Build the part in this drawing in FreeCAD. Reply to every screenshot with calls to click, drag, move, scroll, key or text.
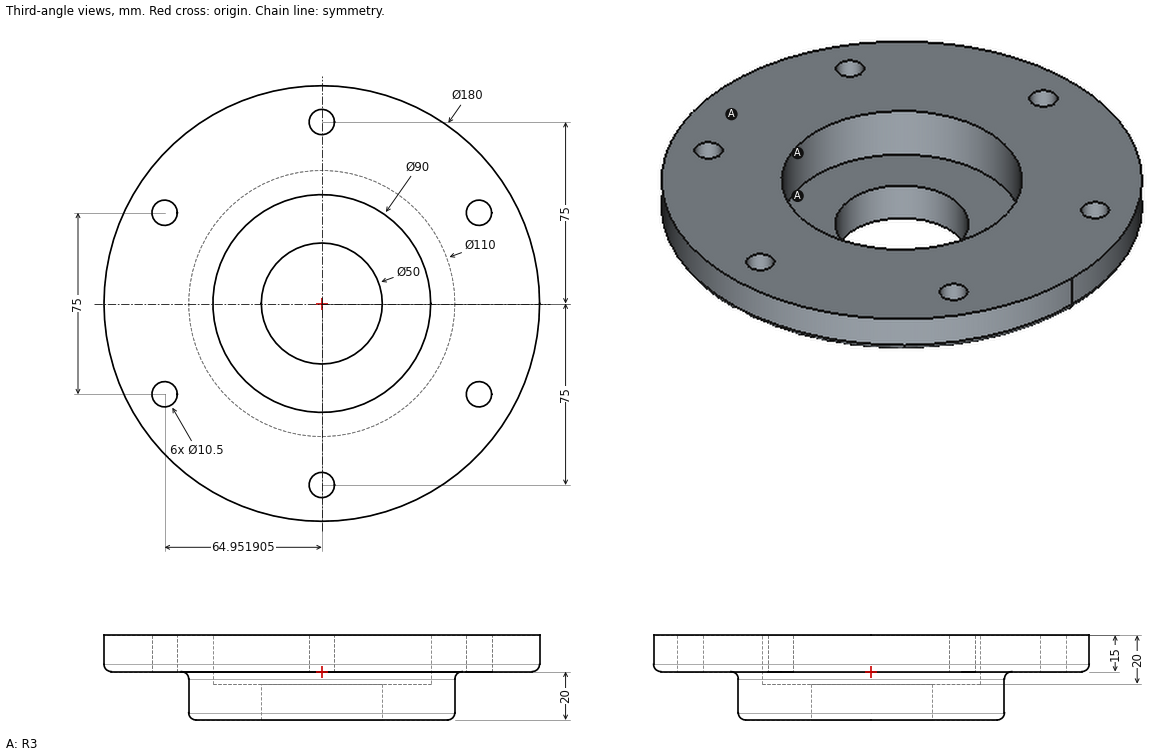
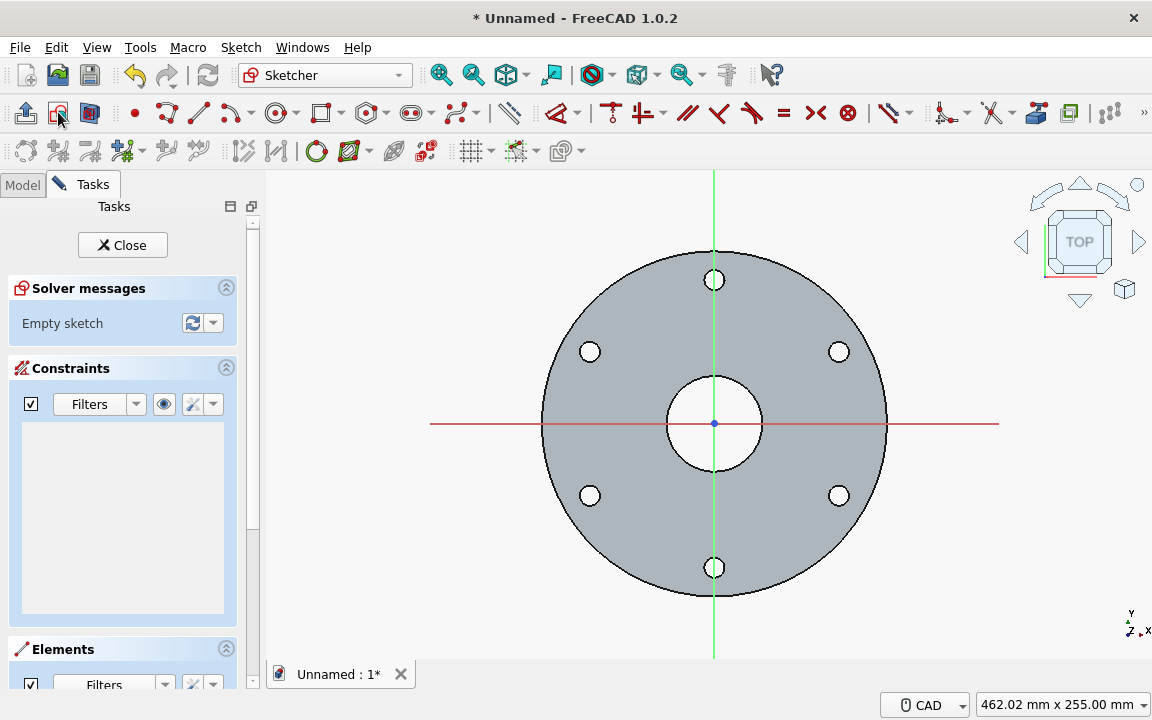
scroll(804, 435, up, 3)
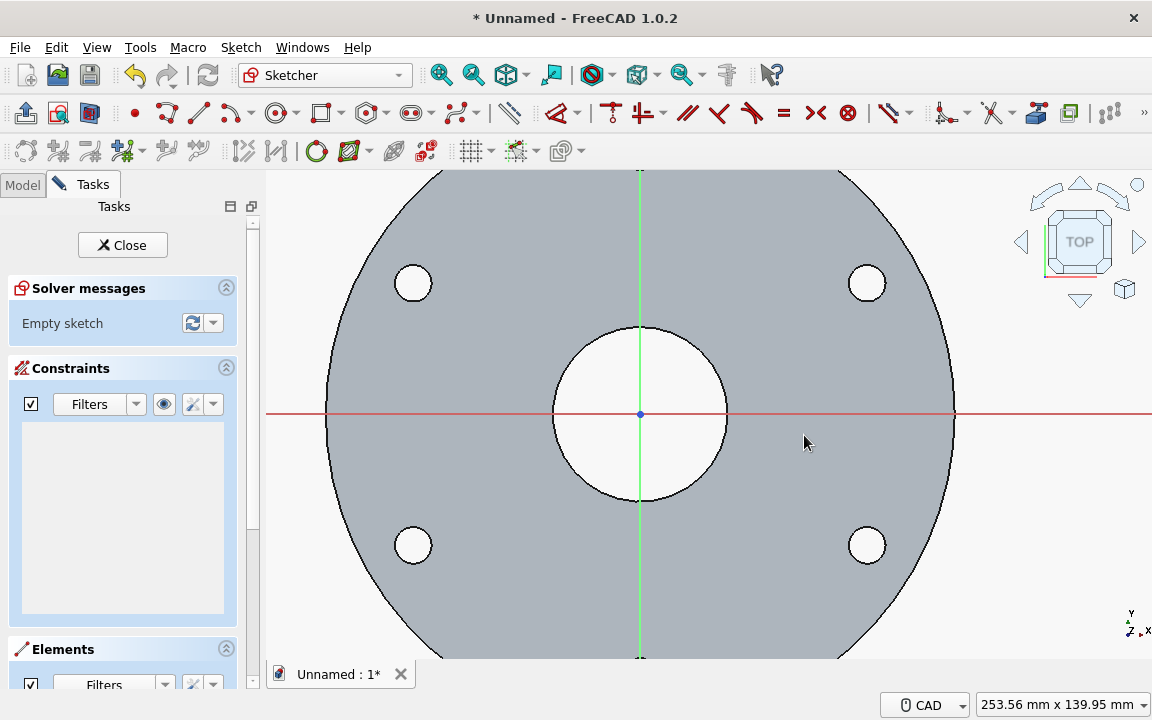
key(g)
key(c)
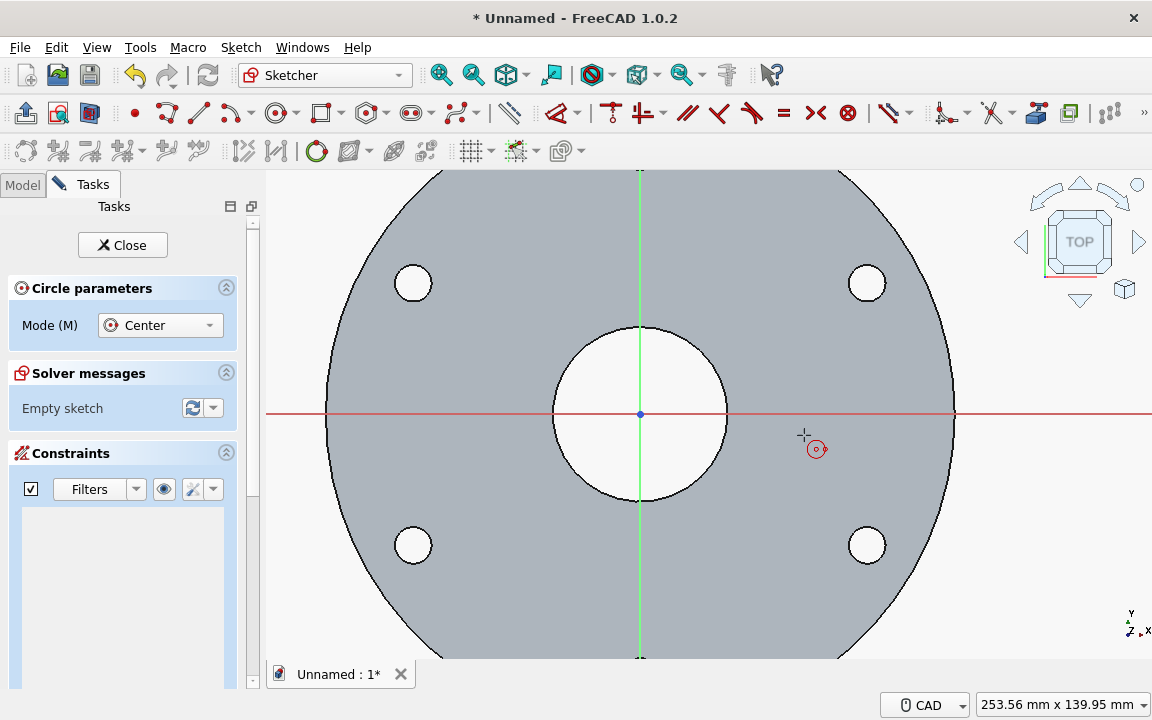
click(640, 414)
move(751, 303)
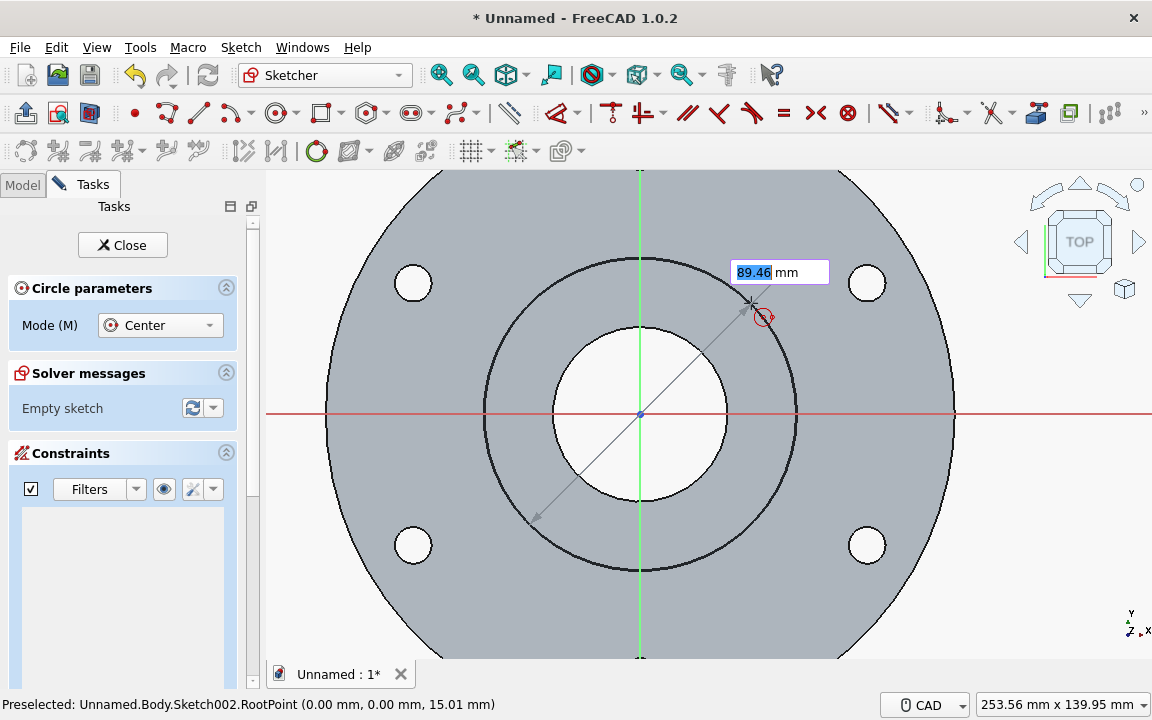
text(90)
key(Return)
key(Escape)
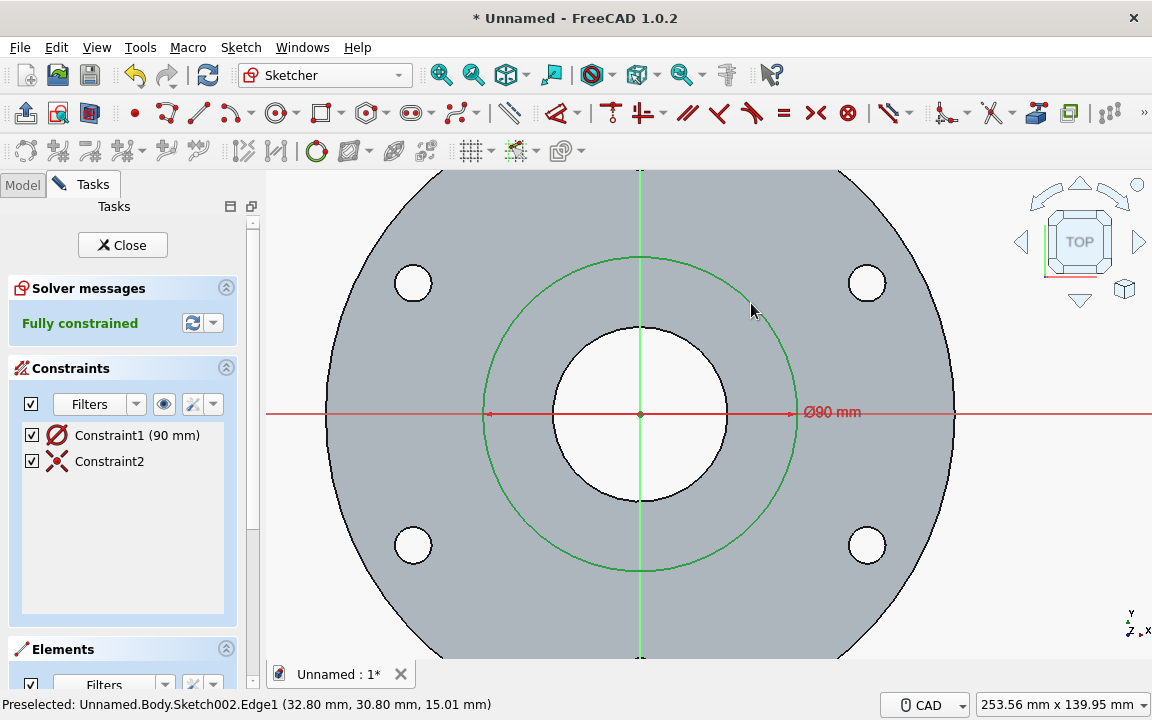
click(123, 245)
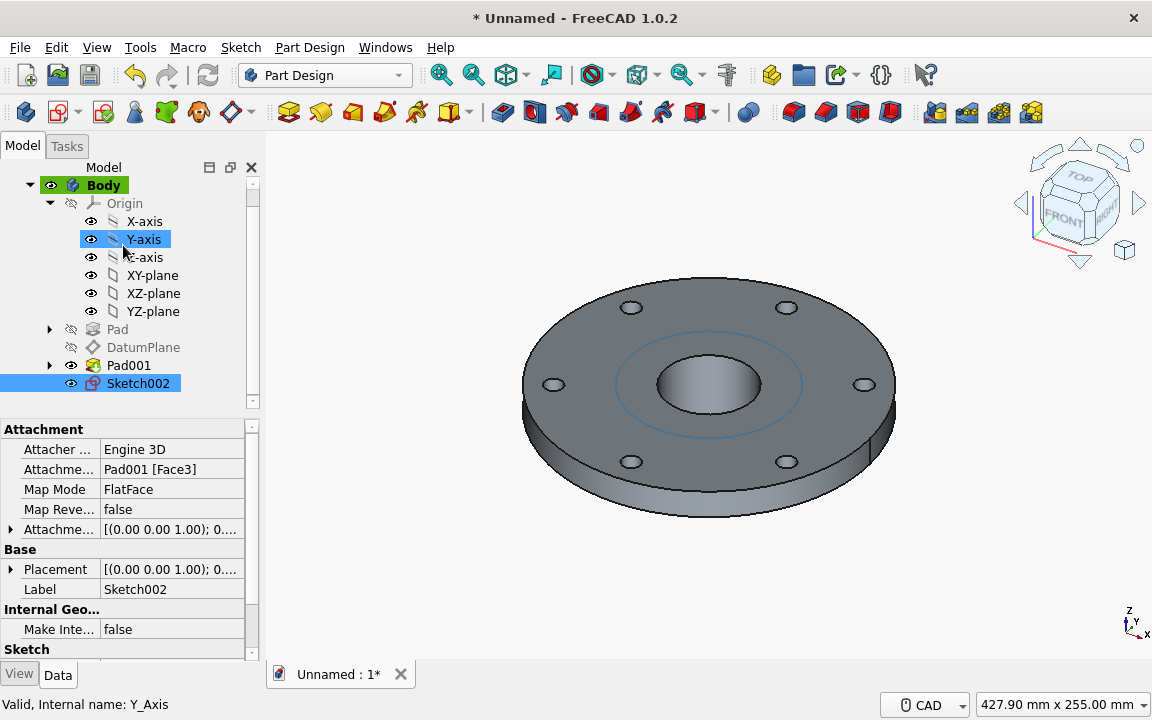
click(504, 112)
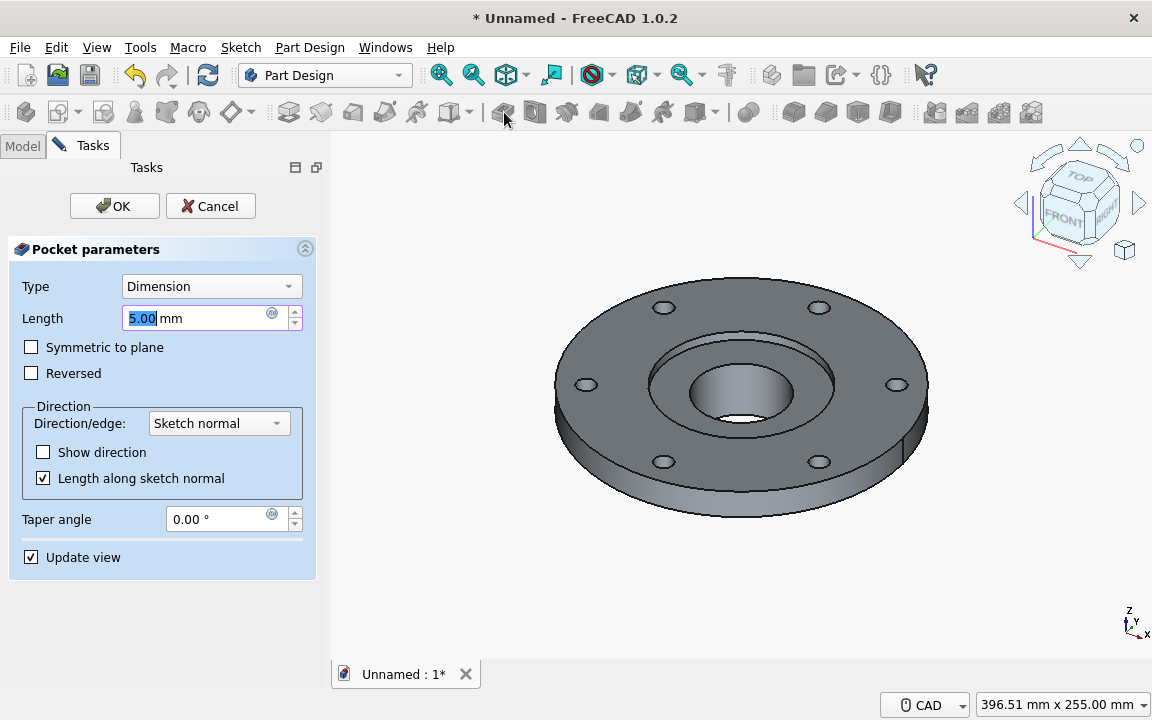
text(20)
key(Tab)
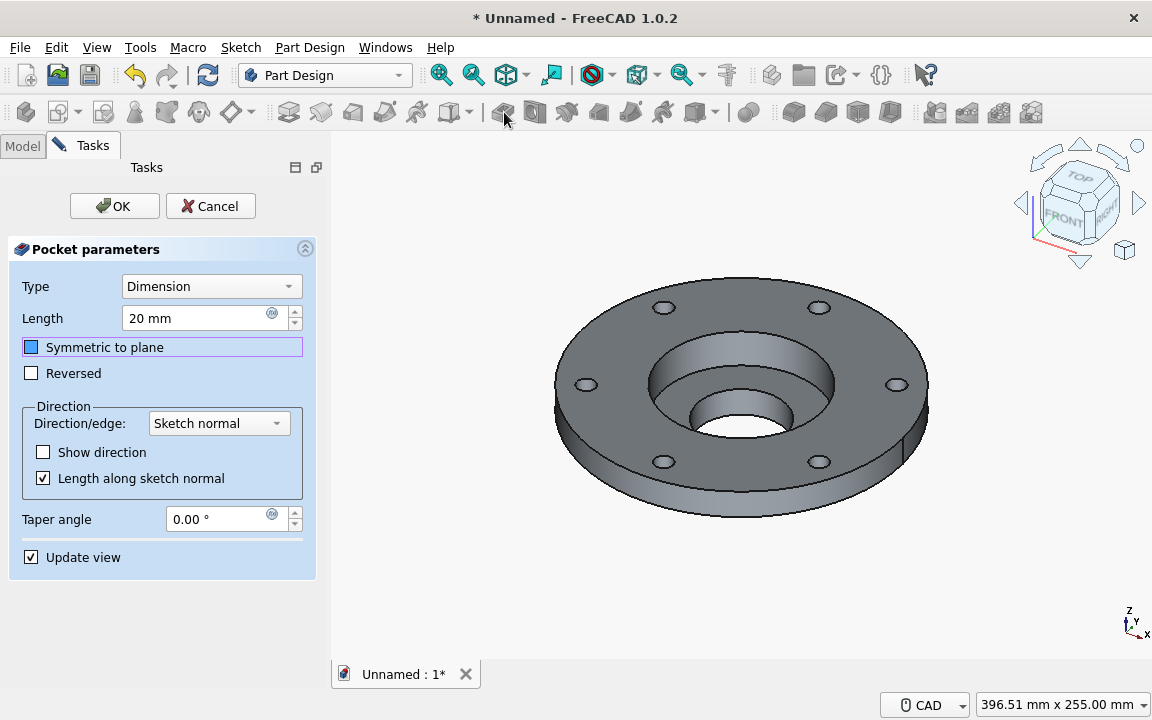
click(115, 206)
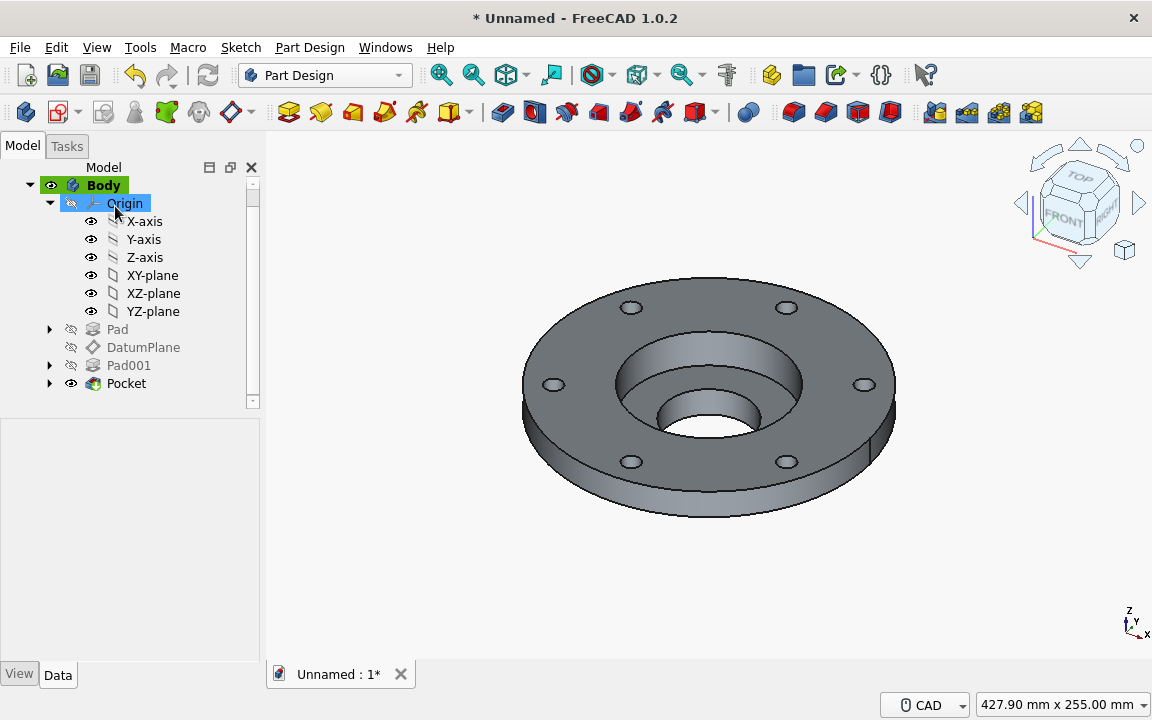
key(0)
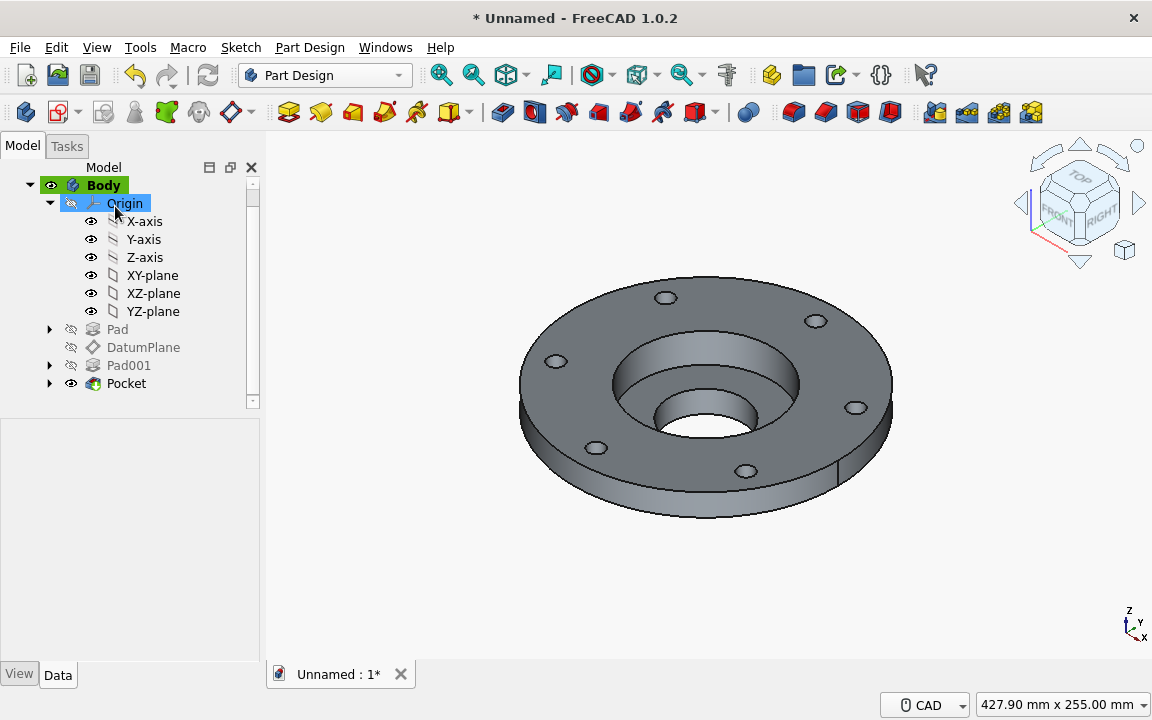
key(2)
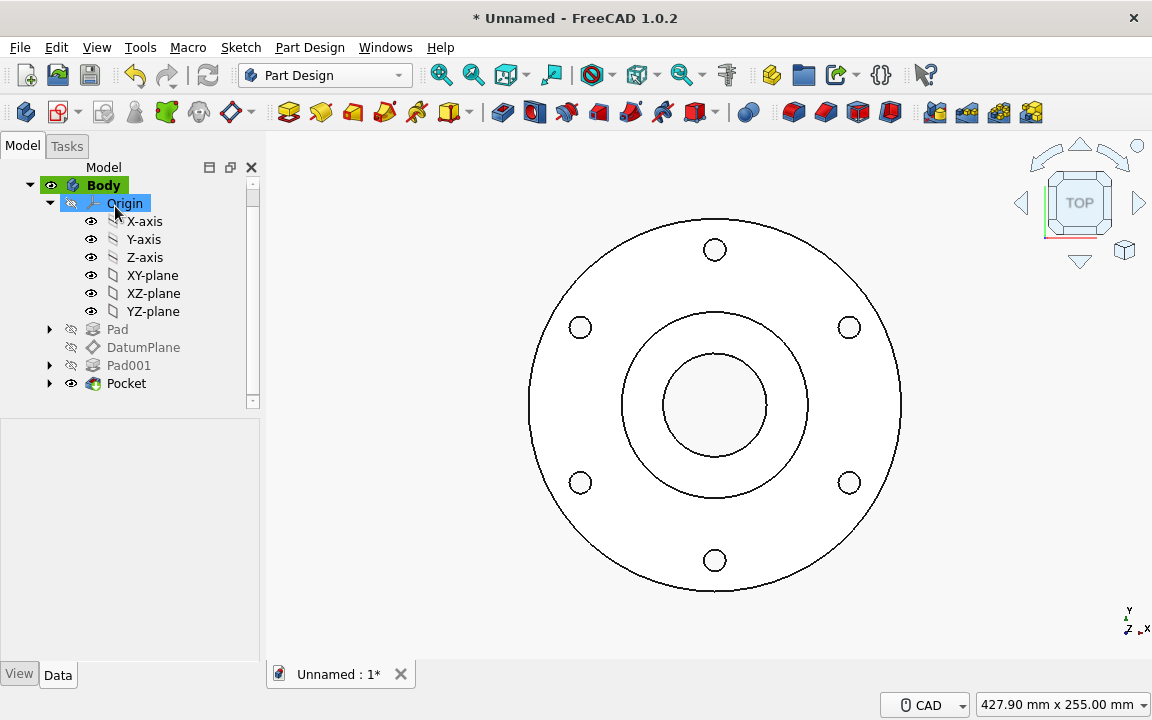
key(1)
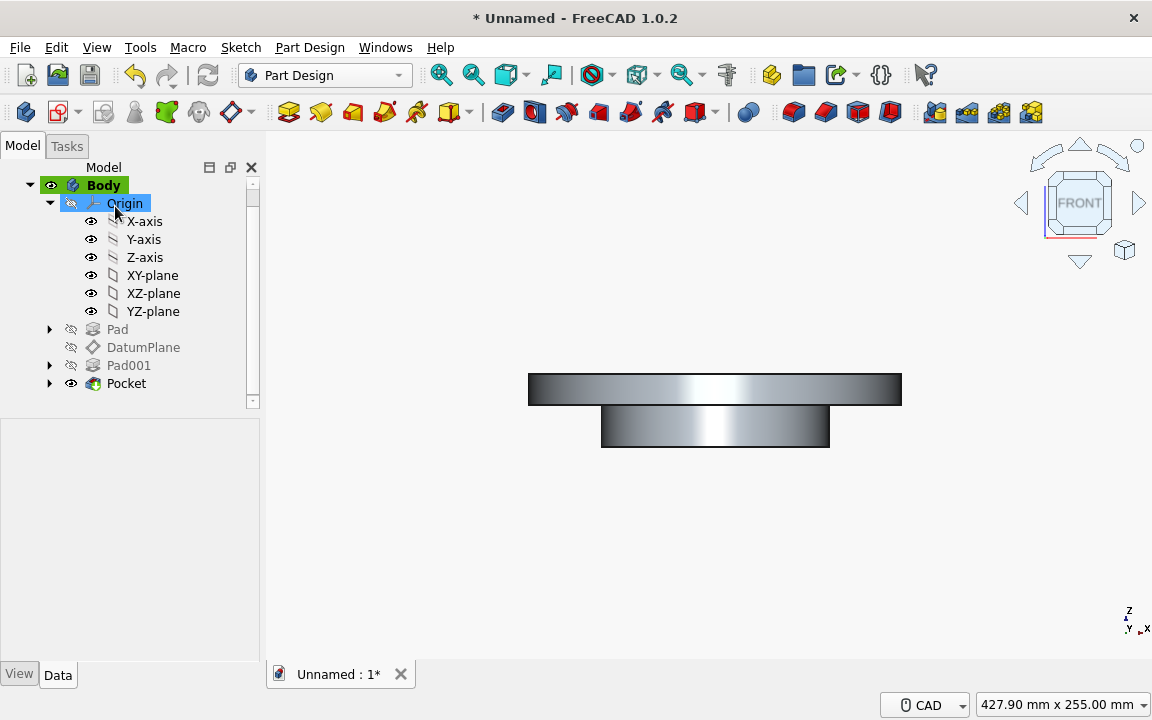
key(v)
key(f)